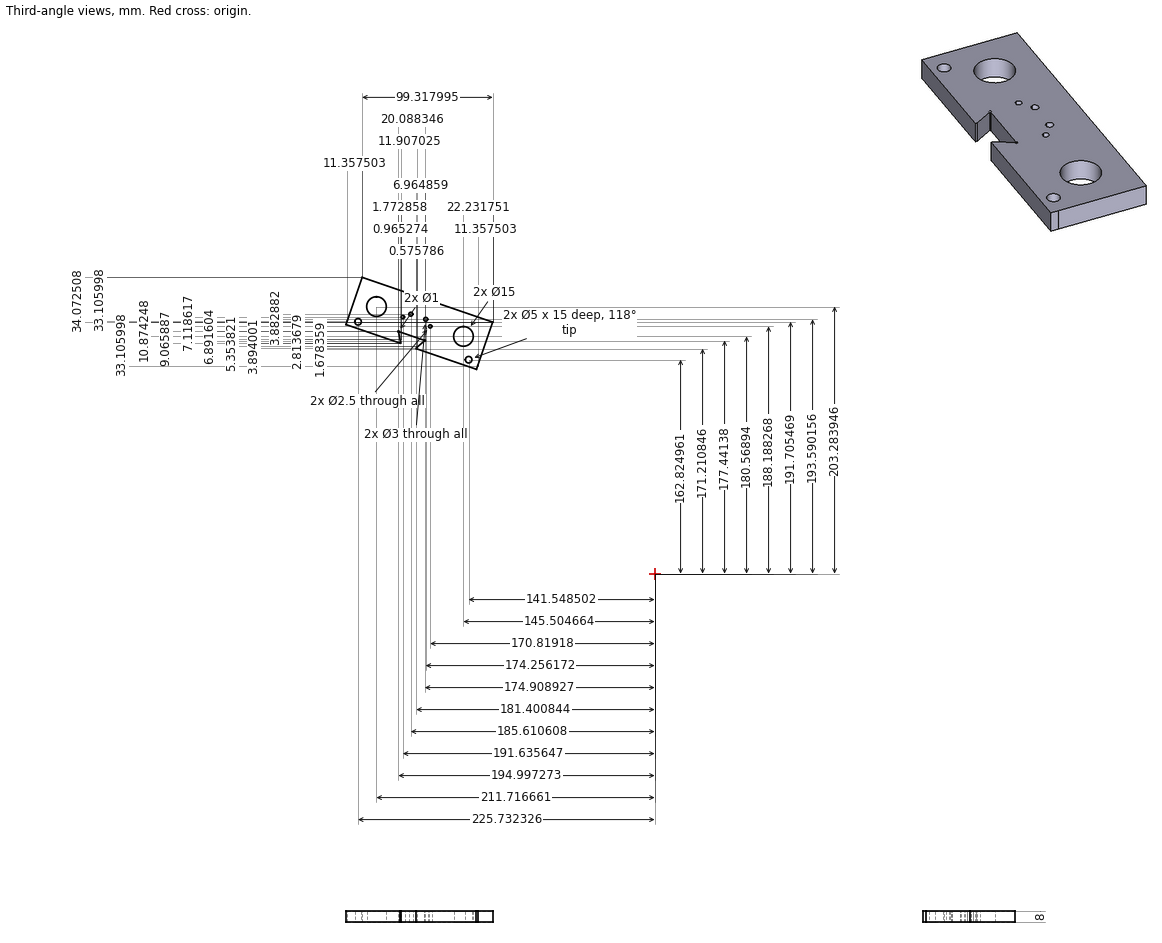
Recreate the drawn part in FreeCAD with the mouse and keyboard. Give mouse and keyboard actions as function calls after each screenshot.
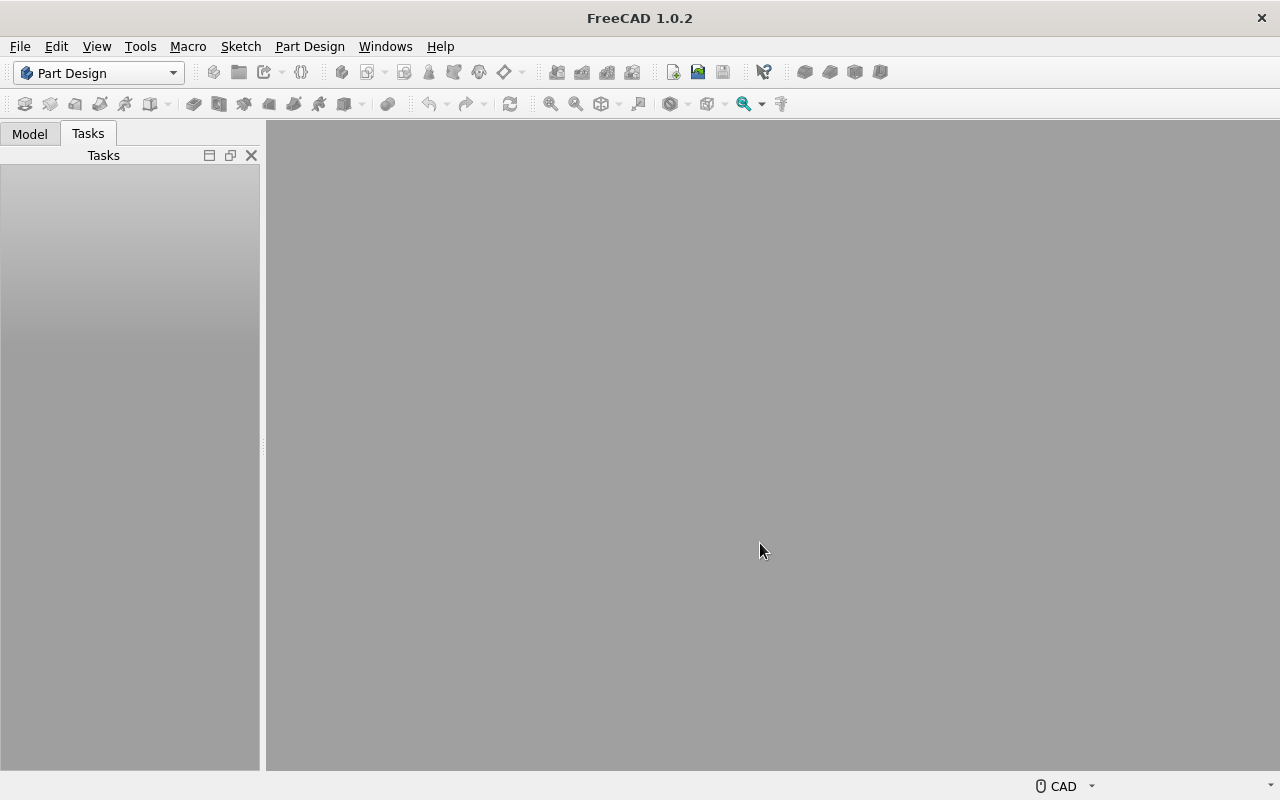
click(673, 72)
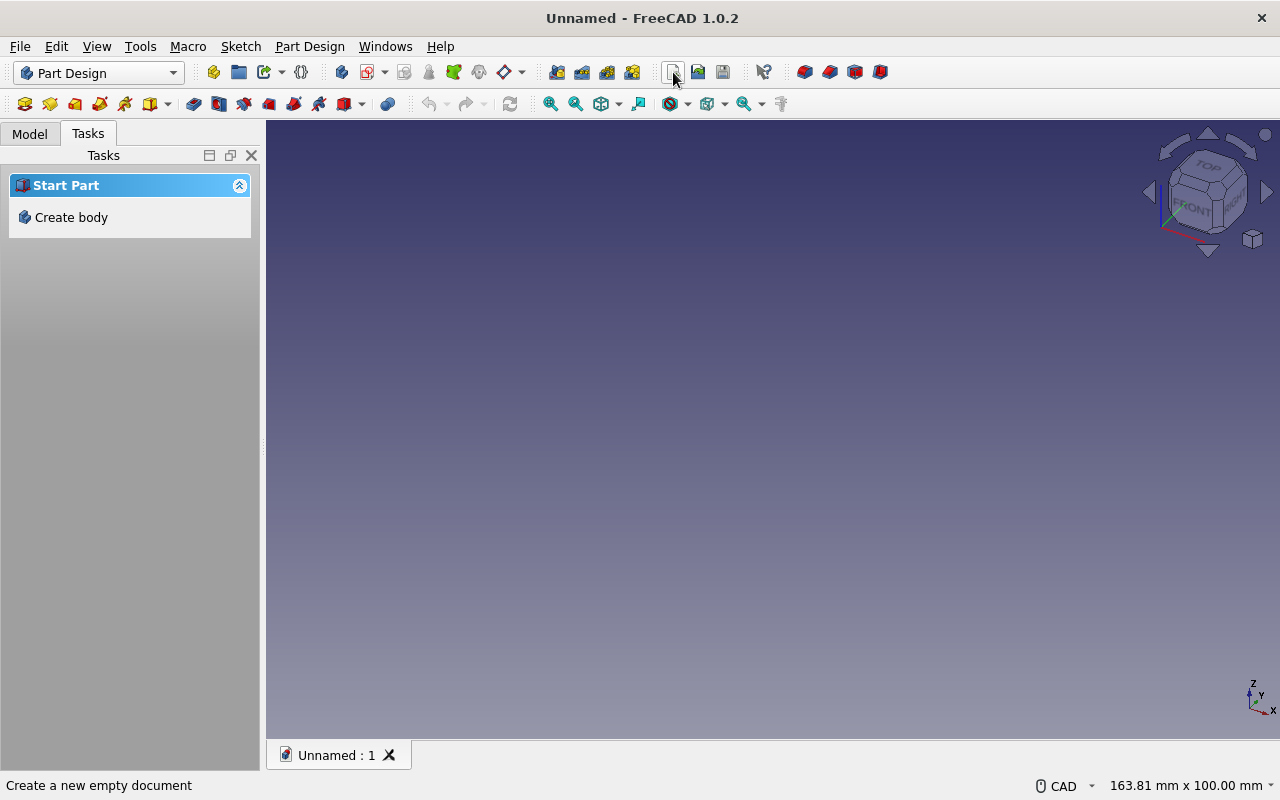
click(366, 72)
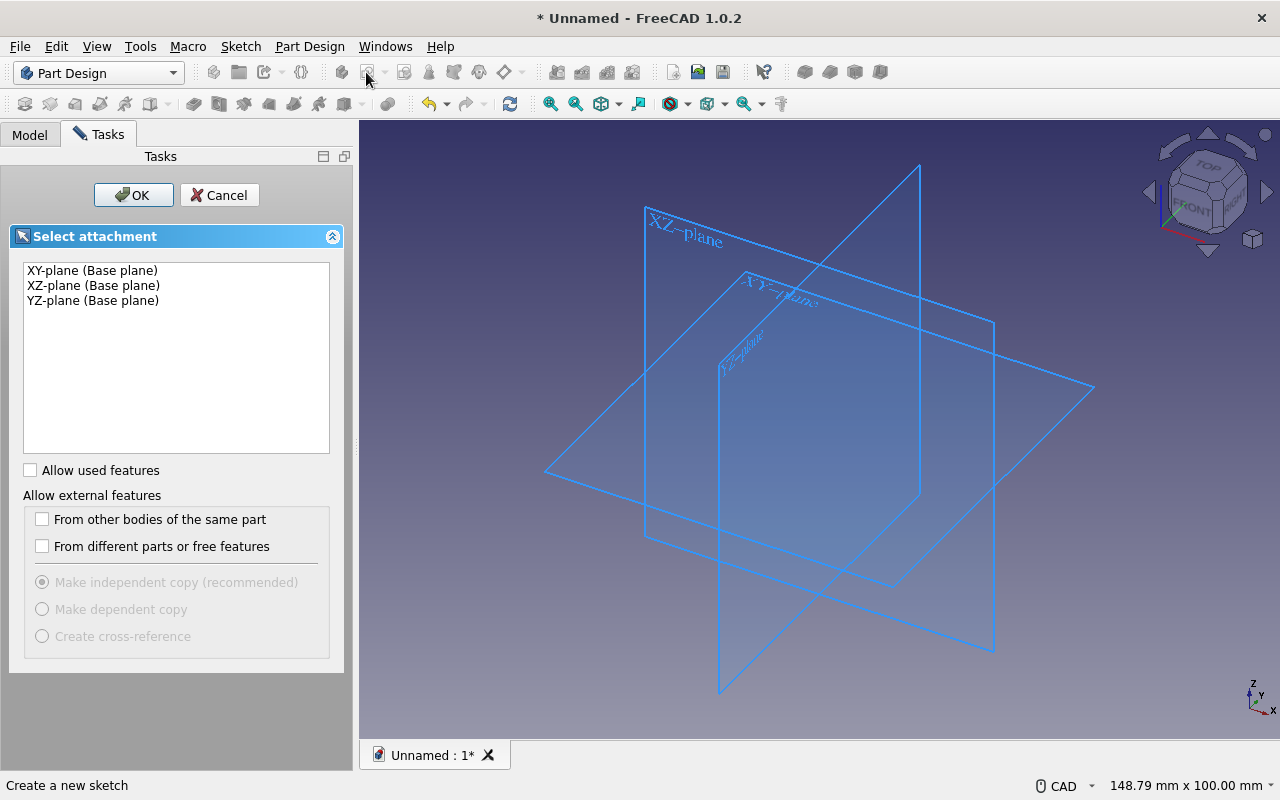
click(84, 270)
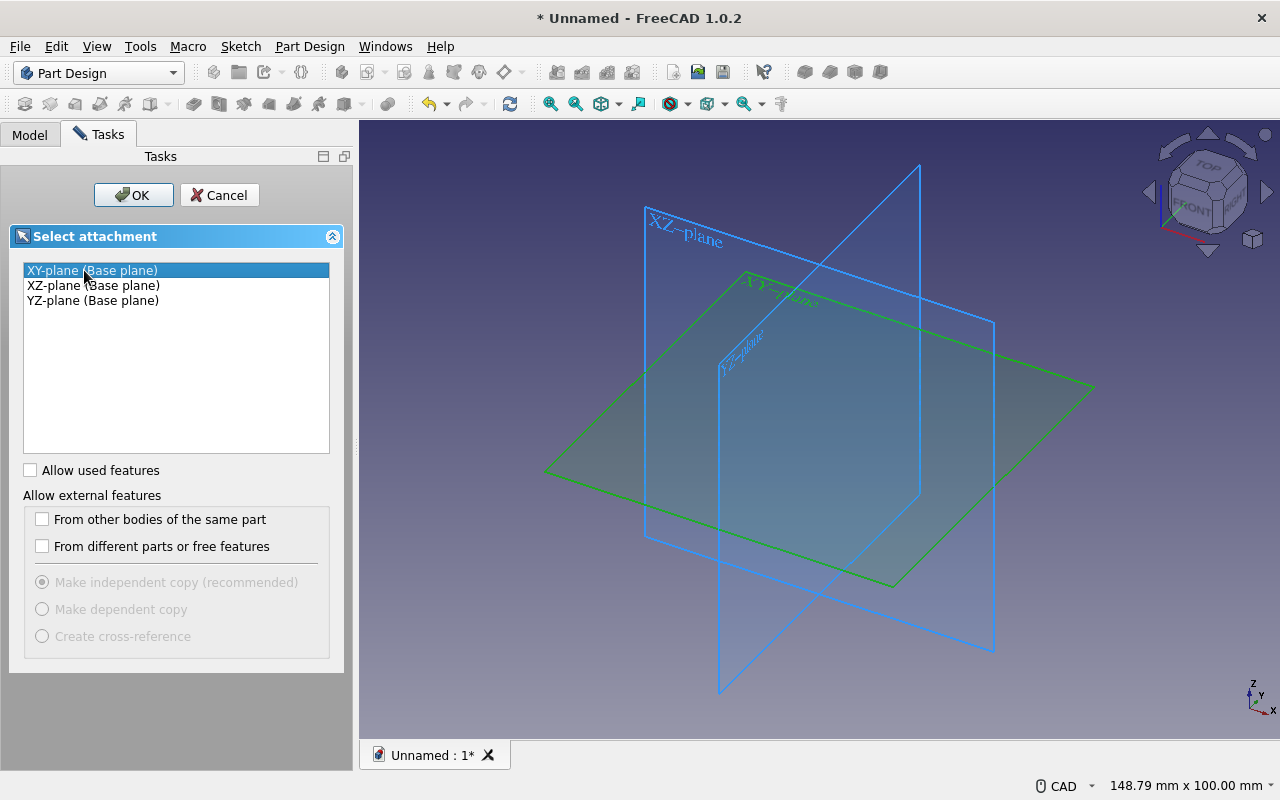
click(134, 195)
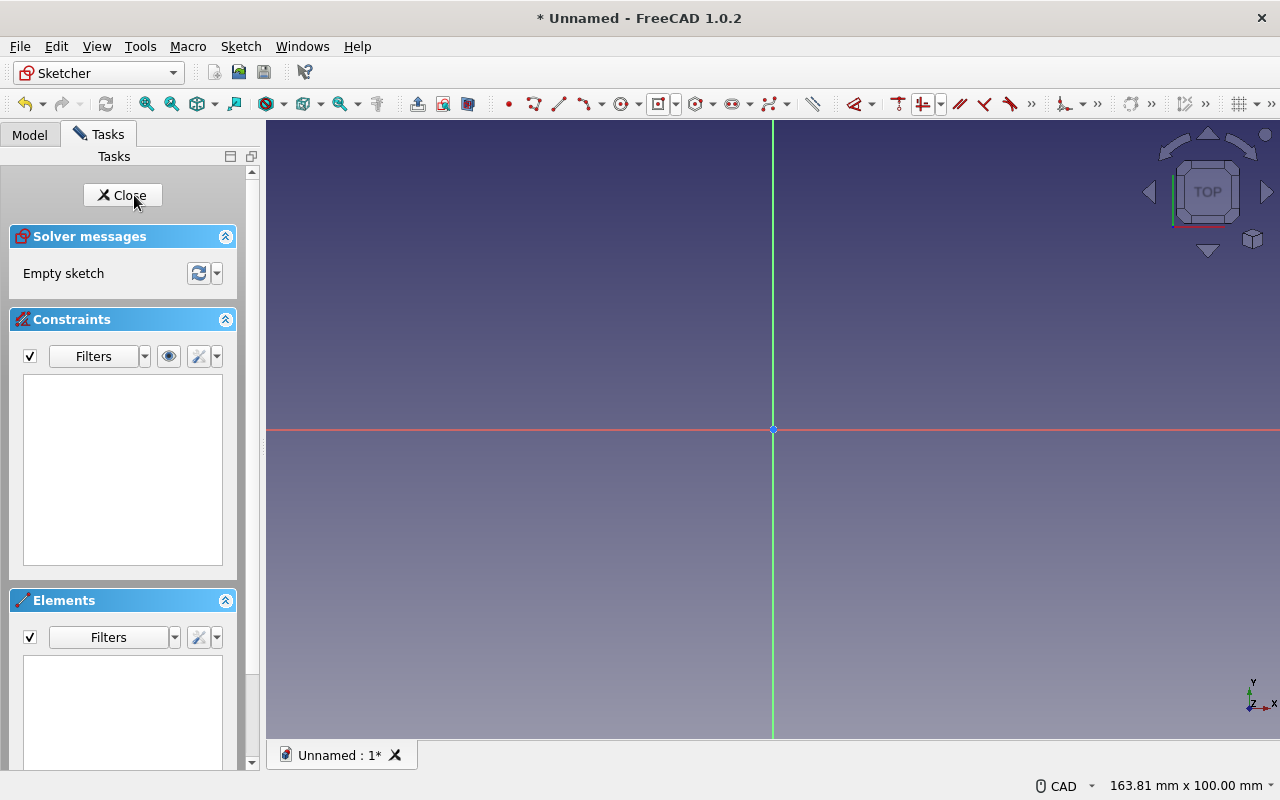
scroll(987, 711, down, 6)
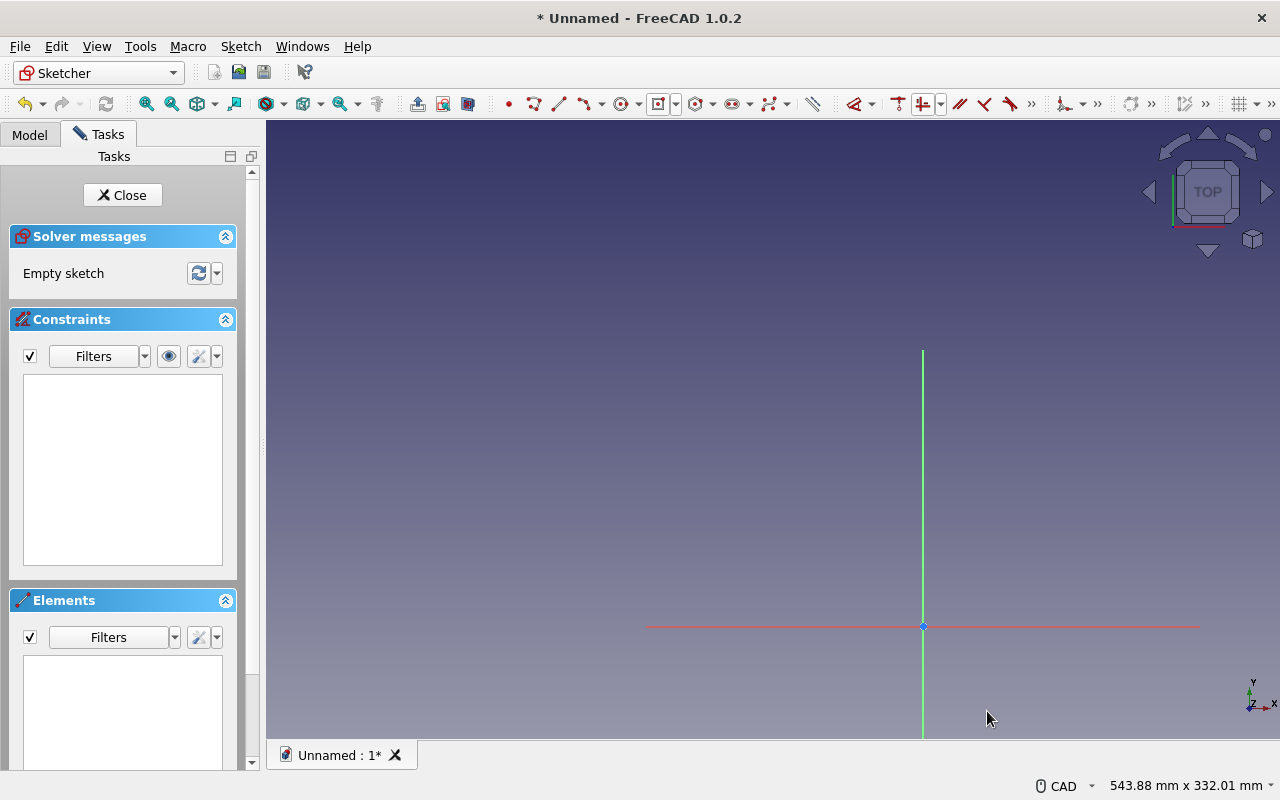
key(g)
key(m)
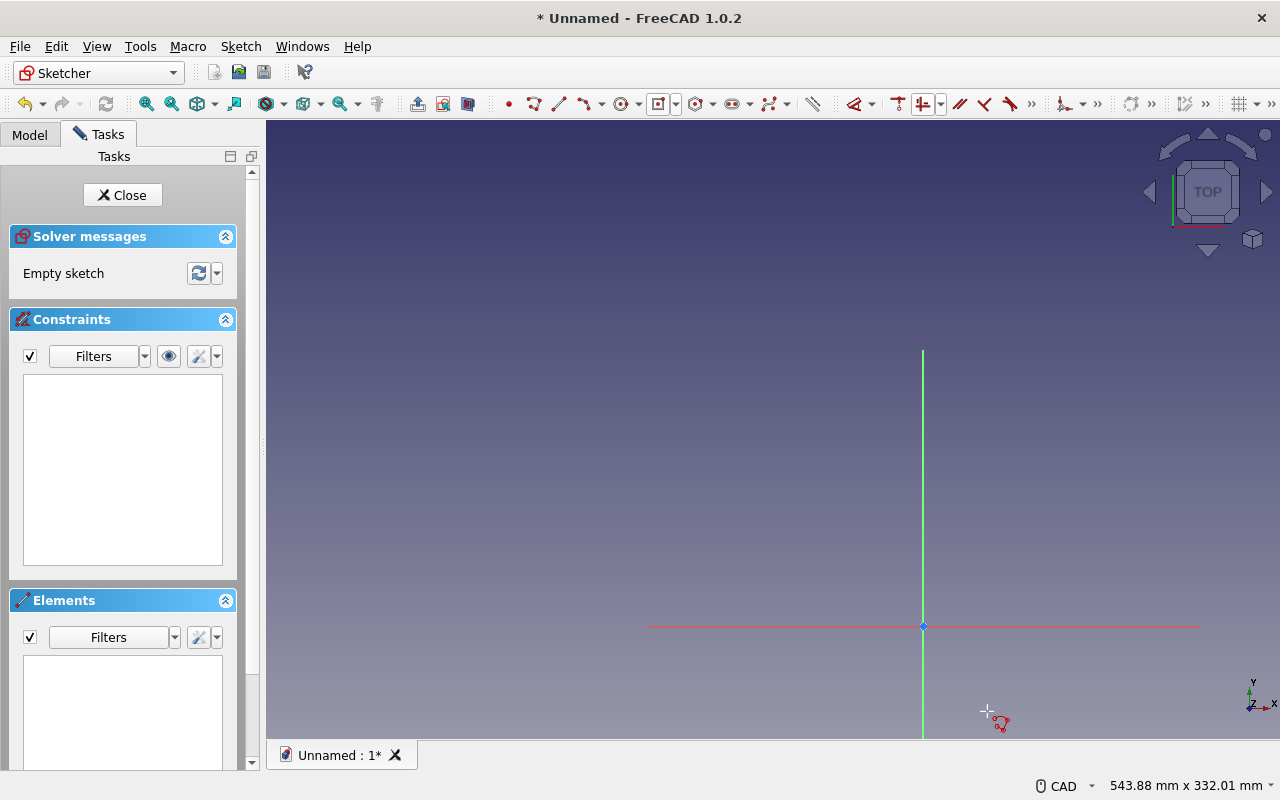
click(672, 332)
click(693, 270)
click(508, 206)
click(487, 268)
click(672, 333)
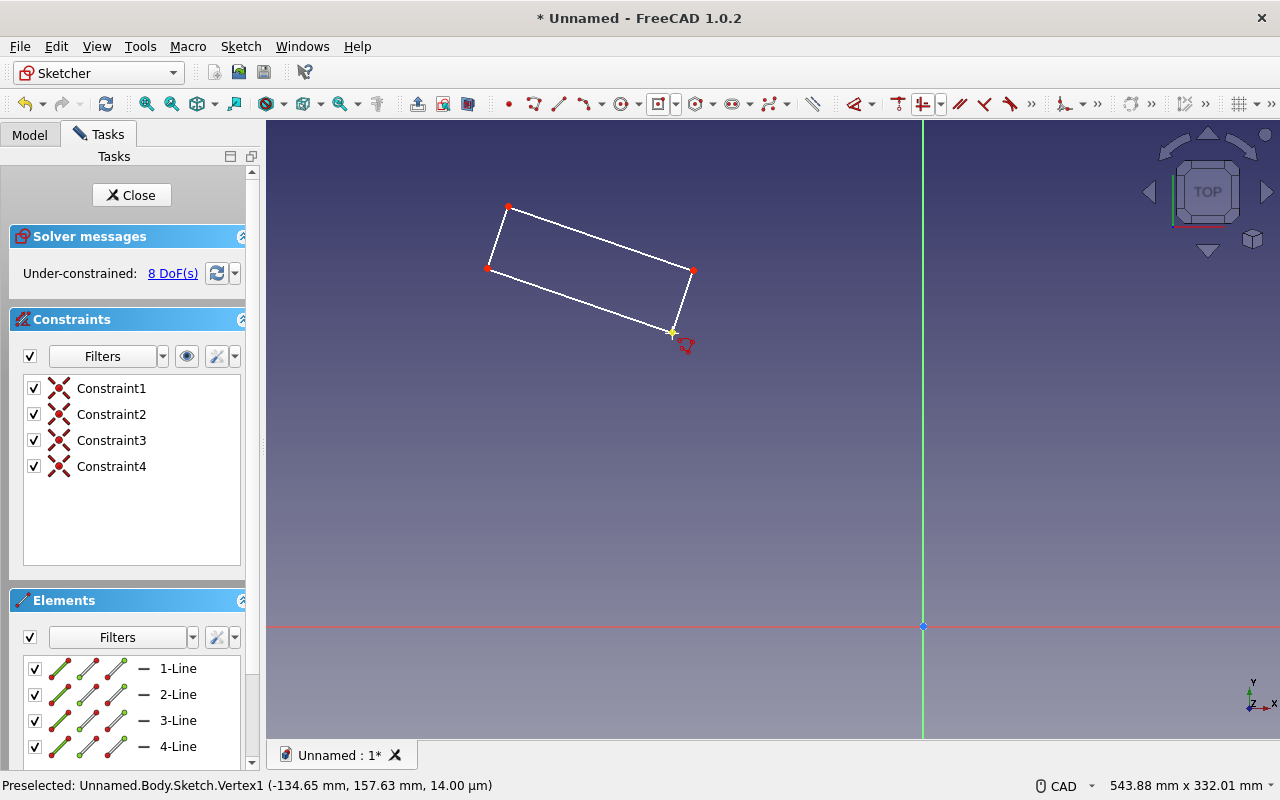
click(620, 104)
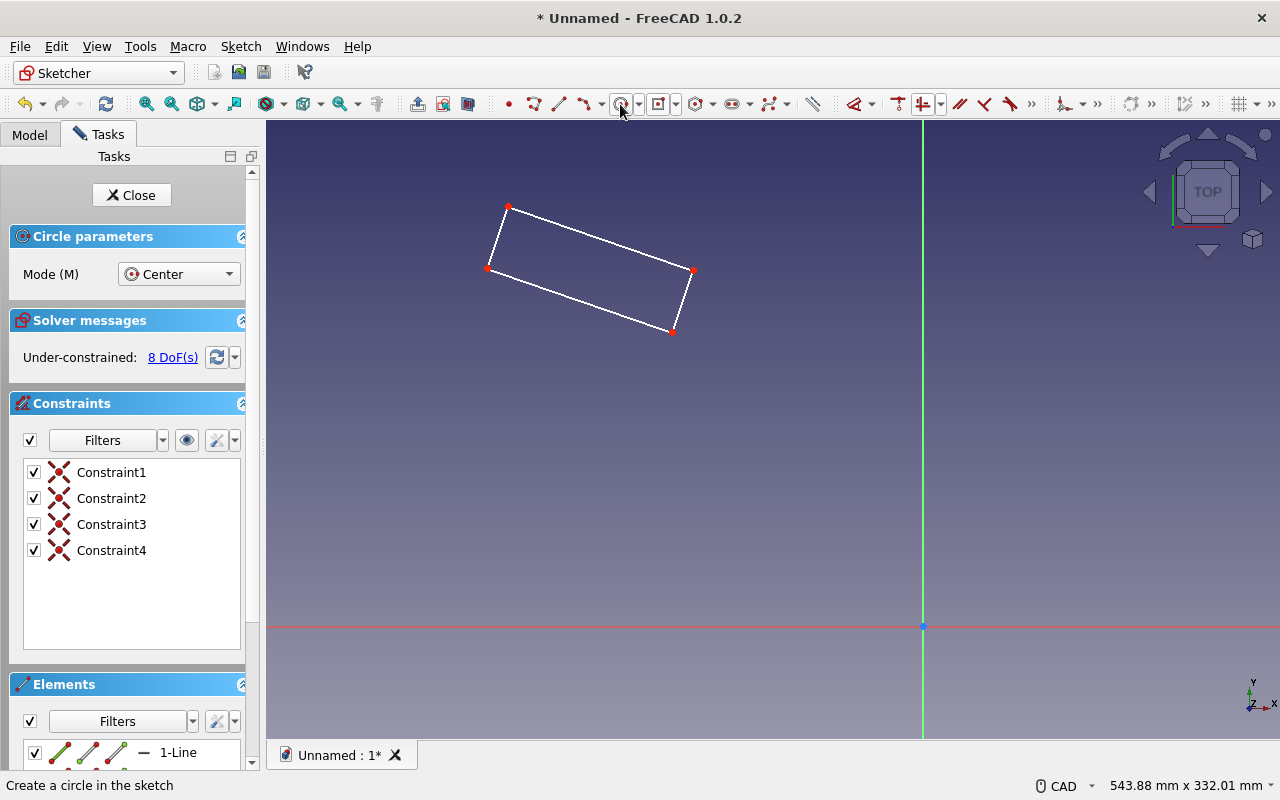
scroll(652, 290, up, 3)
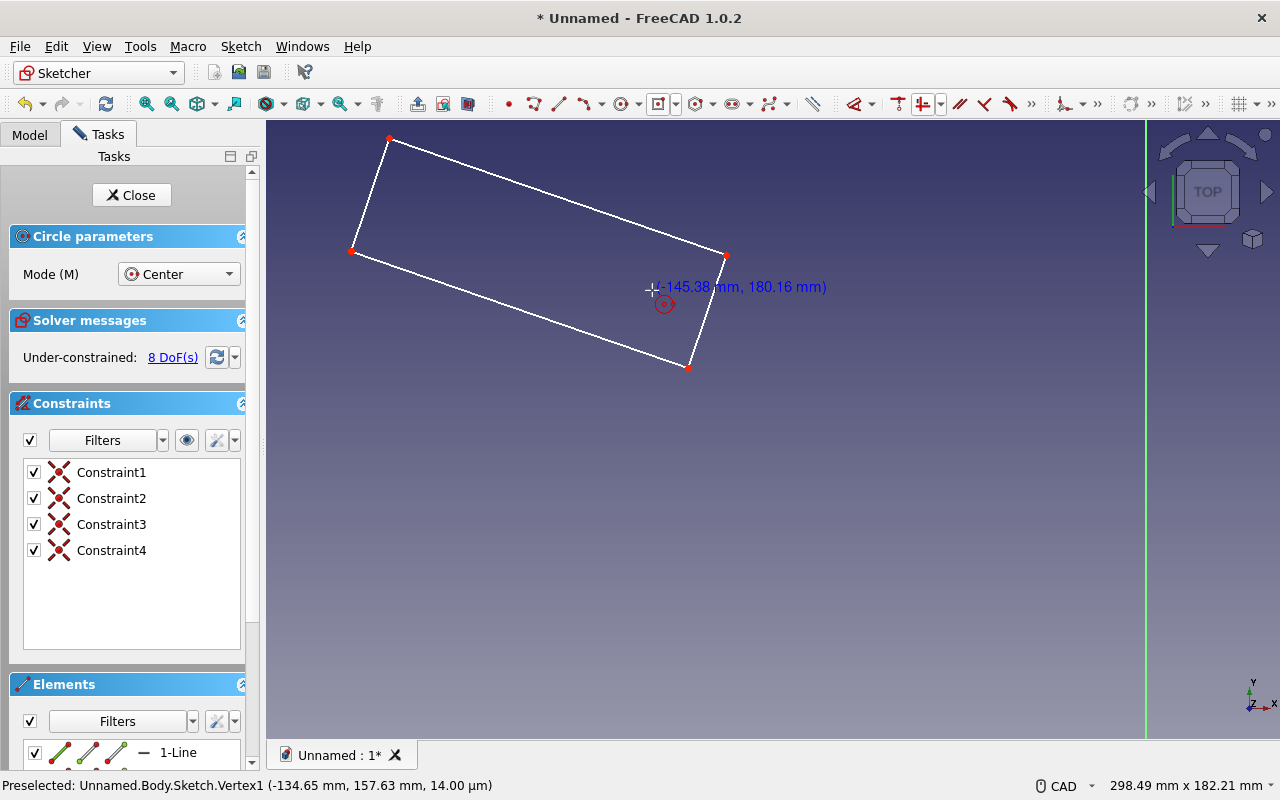
click(651, 290)
click(669, 272)